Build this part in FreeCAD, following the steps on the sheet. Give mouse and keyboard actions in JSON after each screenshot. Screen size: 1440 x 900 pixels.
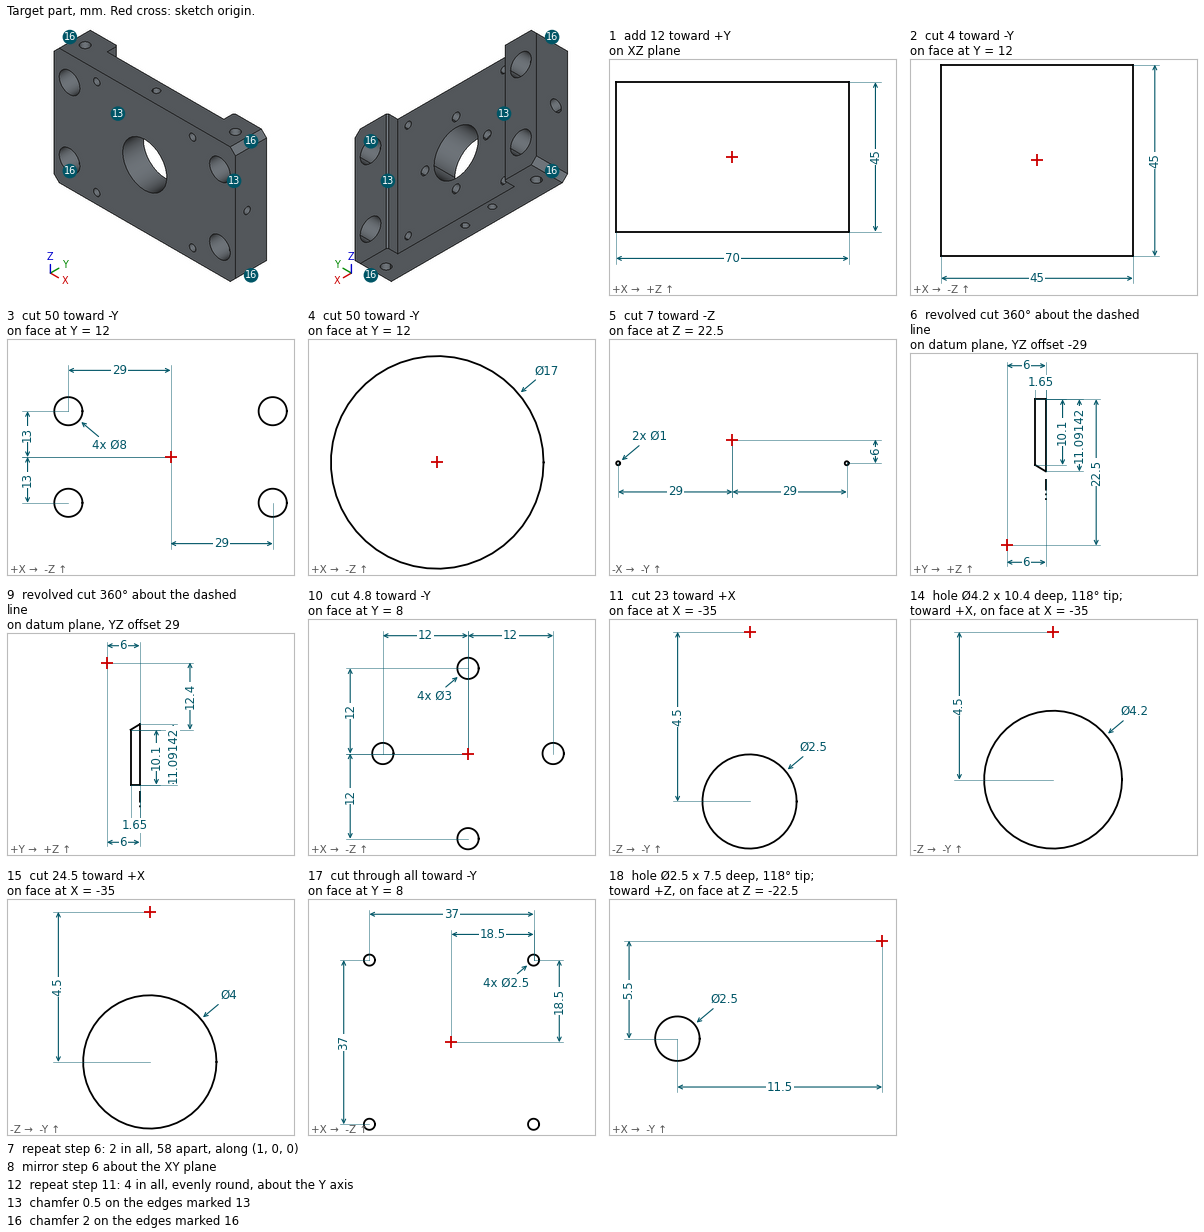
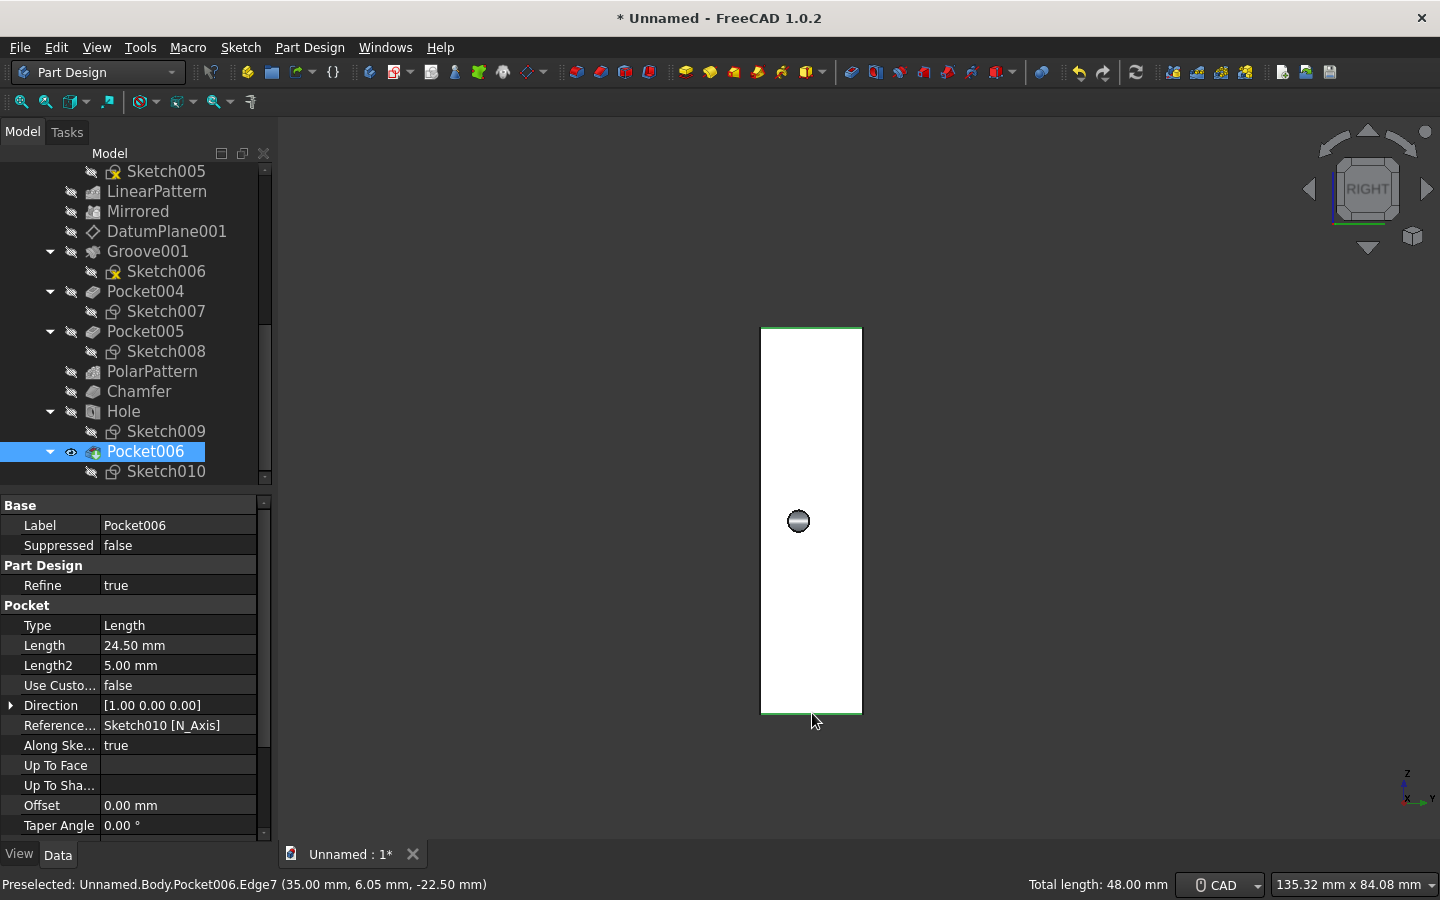
{"action": "left_click", "coordinate": [602, 72]}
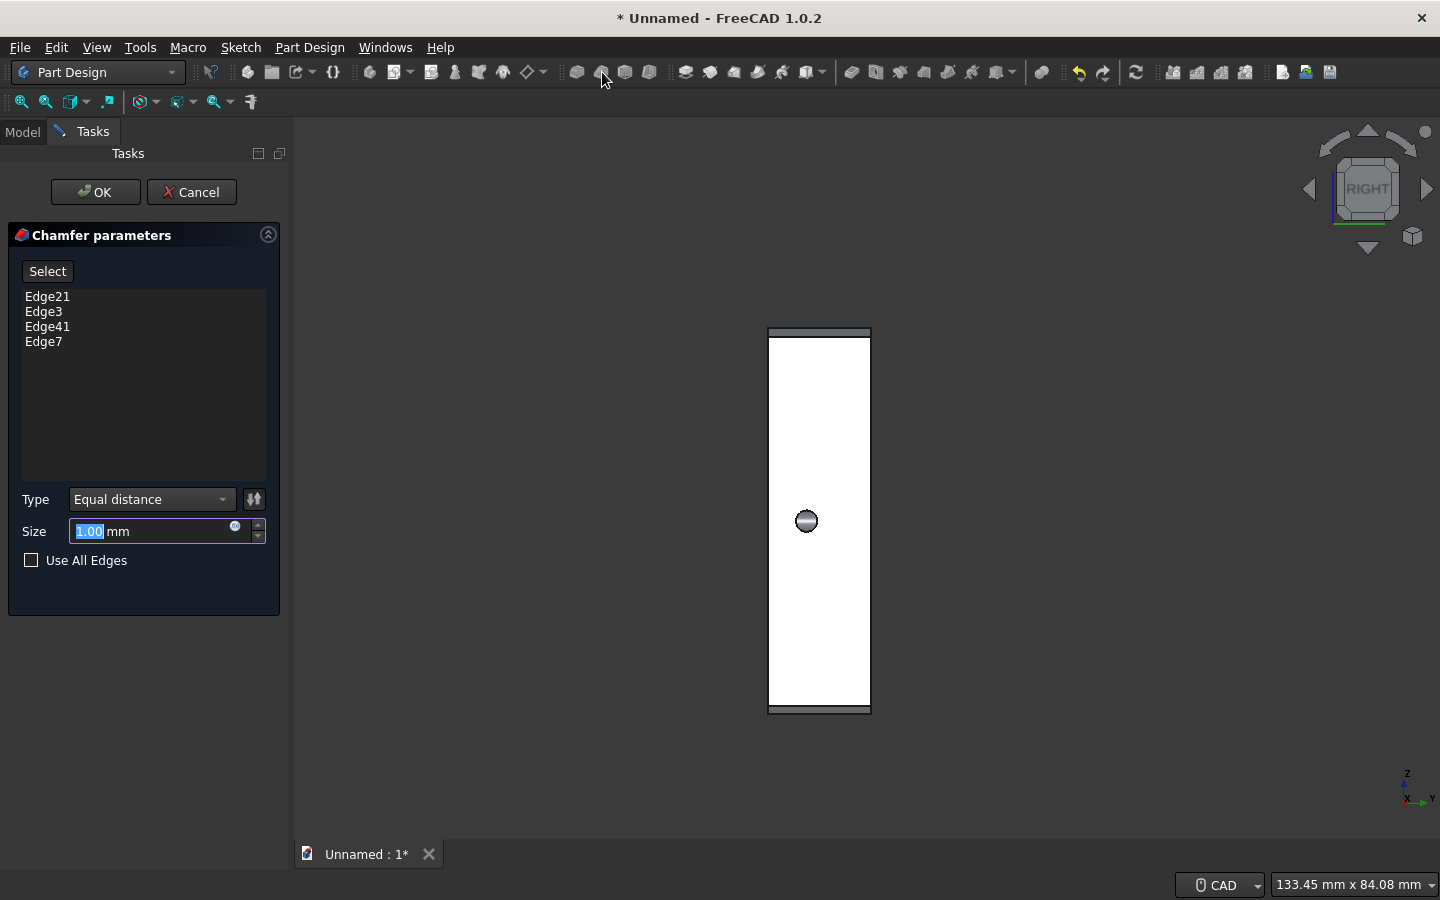
{"action": "type", "text": "2"}
{"action": "key", "text": "Tab"}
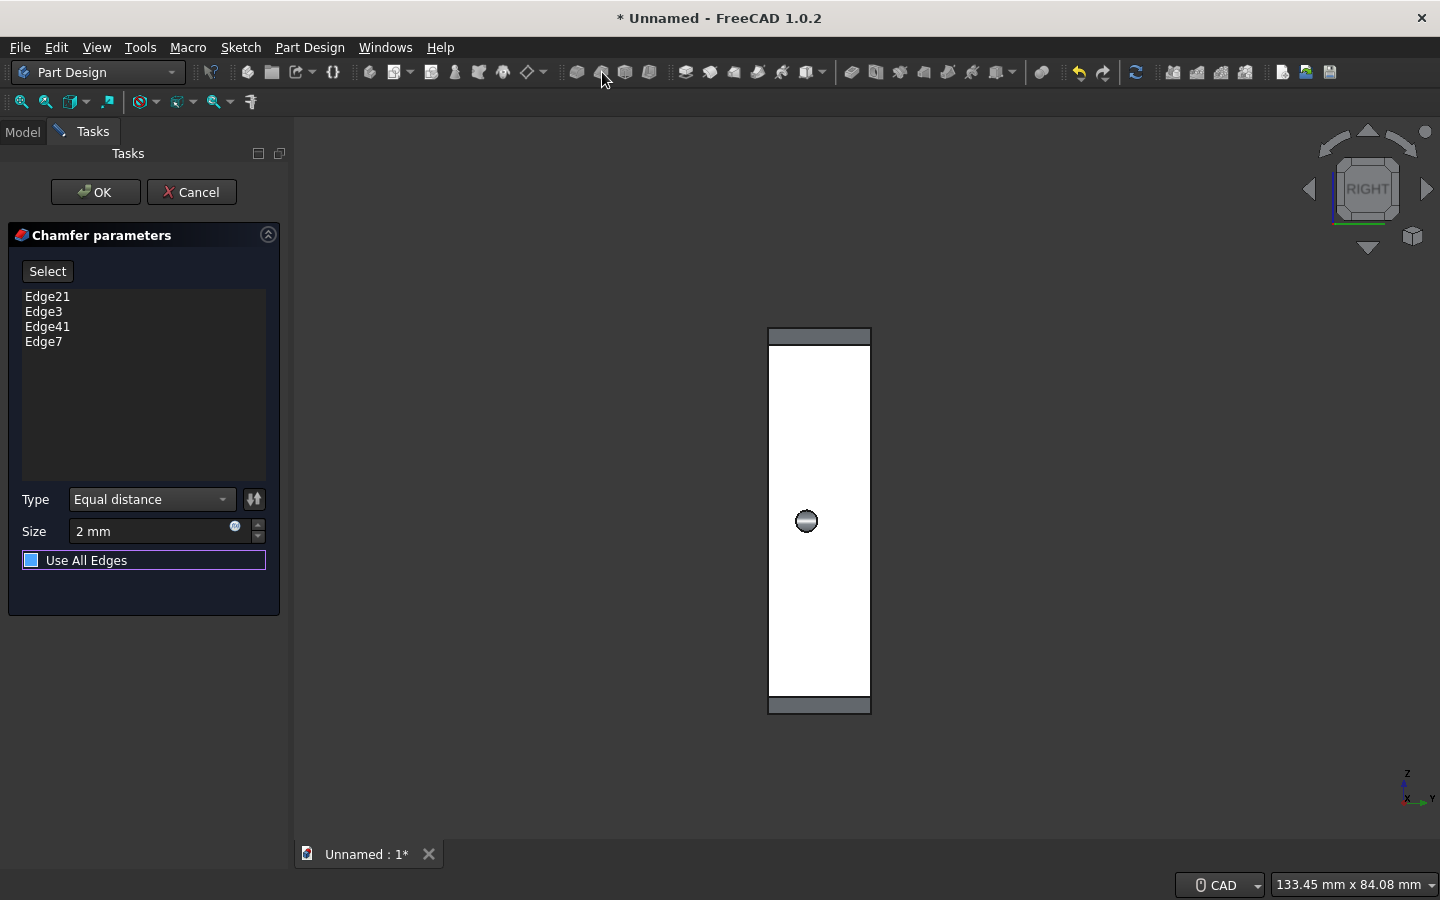
{"action": "left_click", "coordinate": [96, 192]}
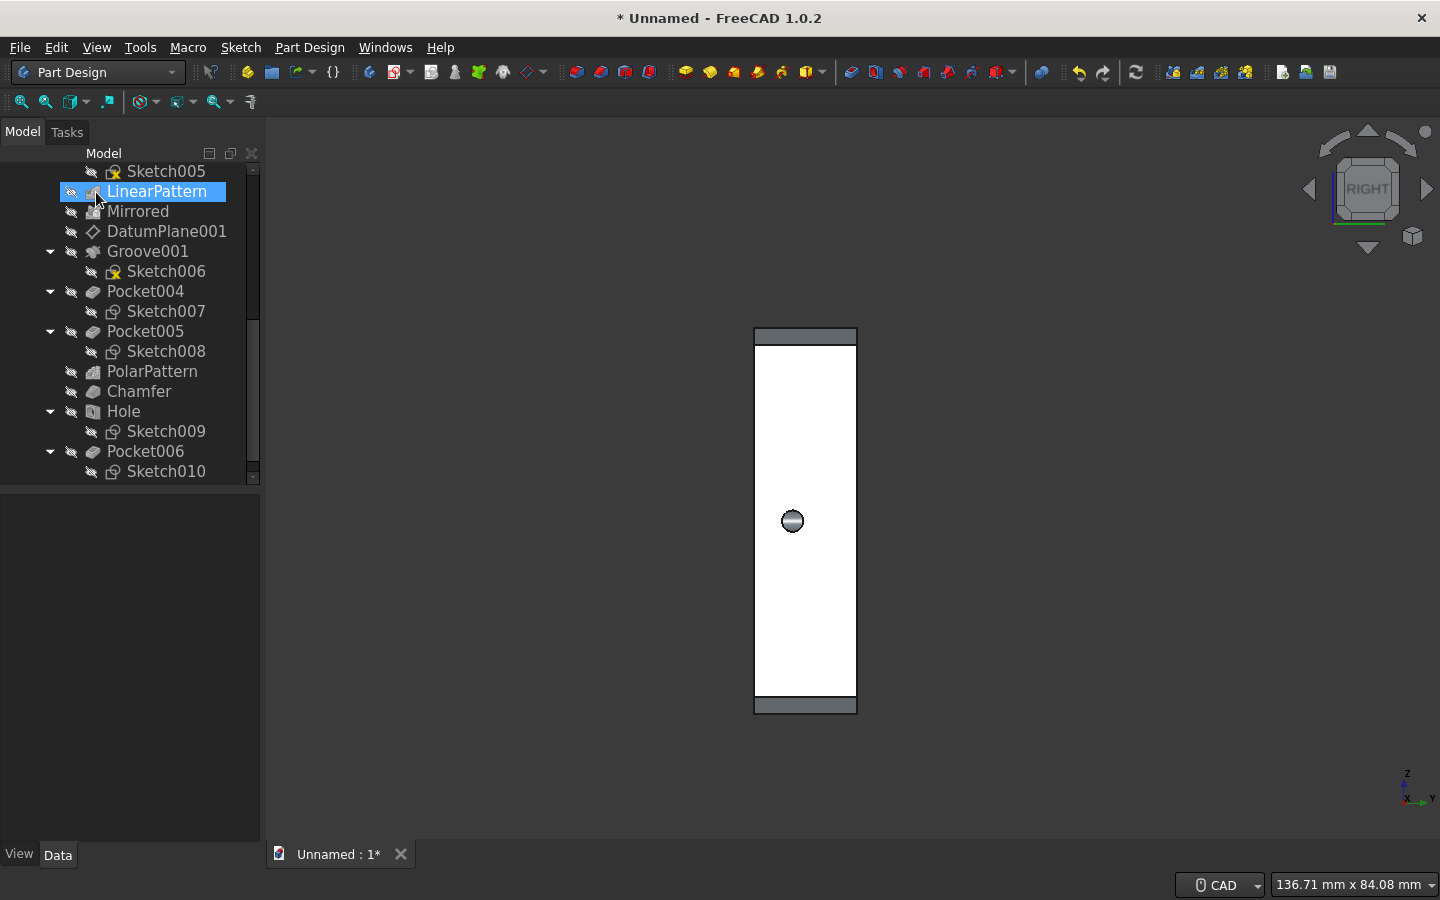
{"action": "key", "text": "4"}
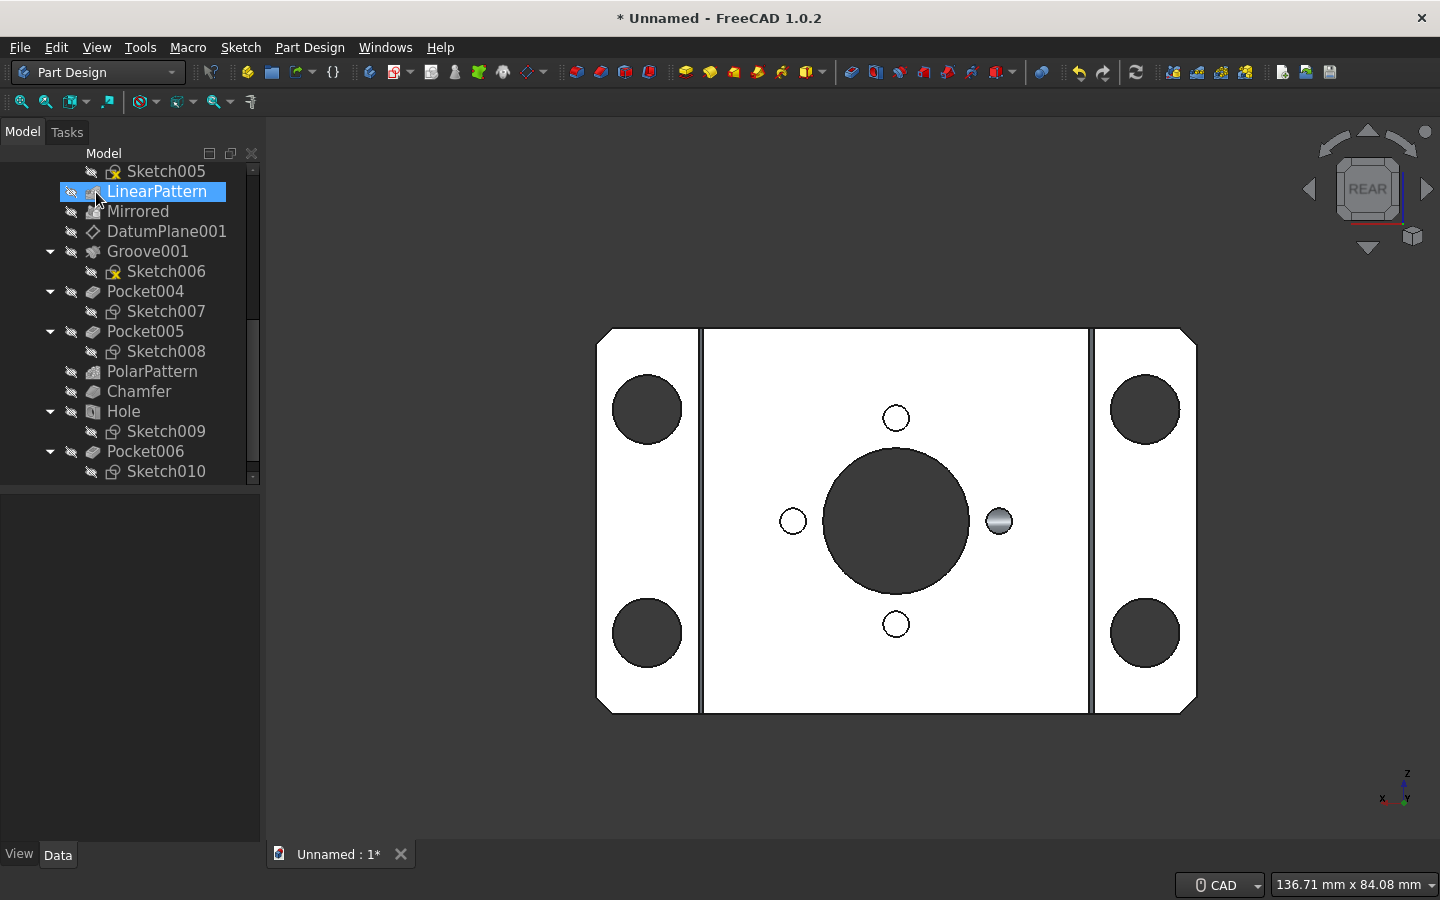
{"action": "left_click", "coordinate": [786, 410]}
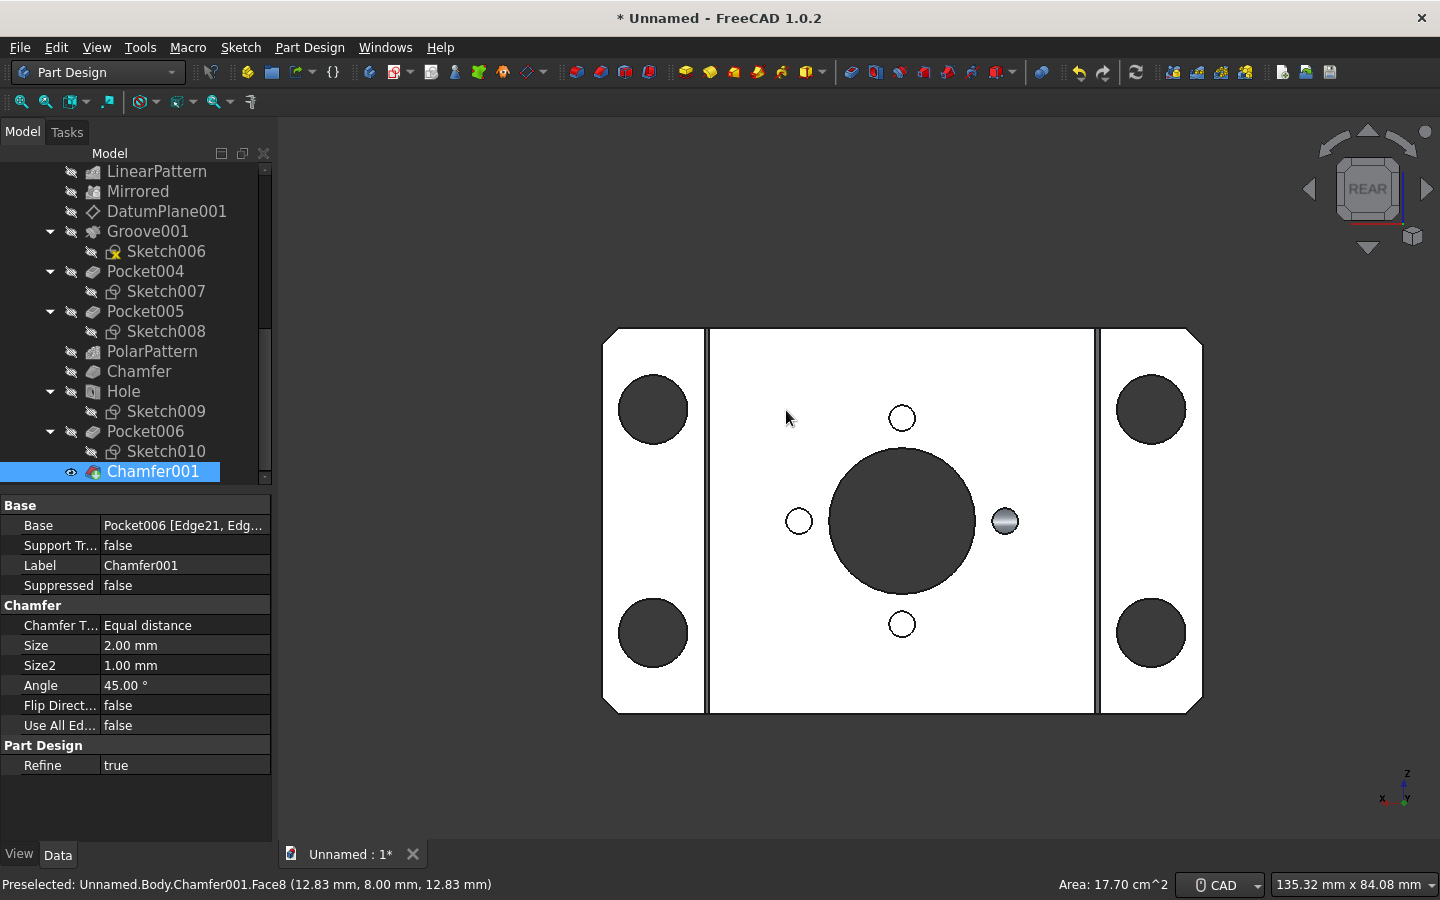
{"action": "left_click", "coordinate": [394, 72]}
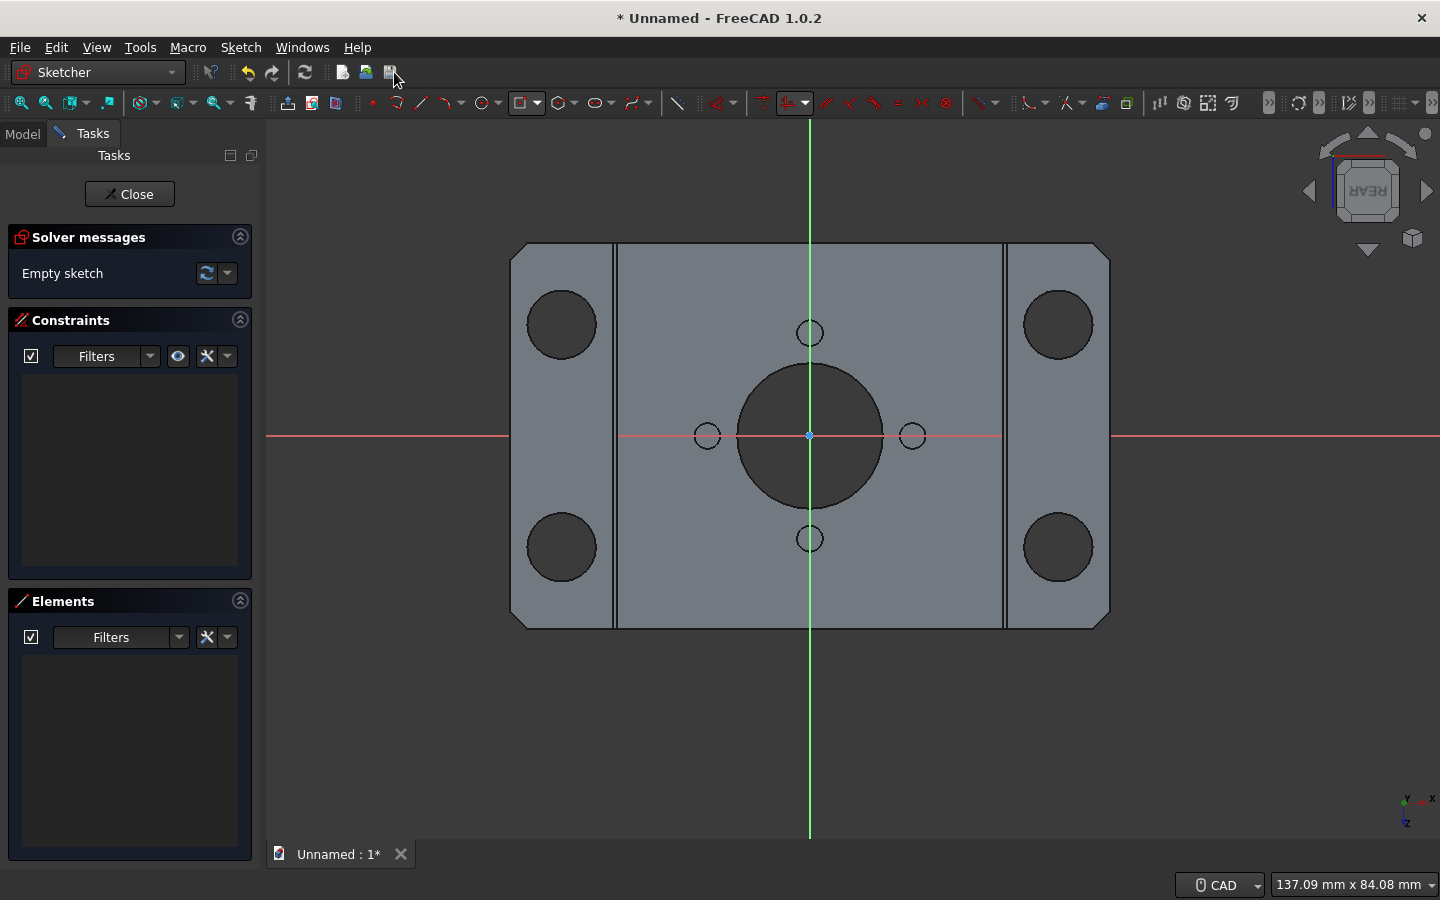
{"action": "scroll", "coordinate": [862, 349], "scroll_direction": "up", "scroll_amount": 2}